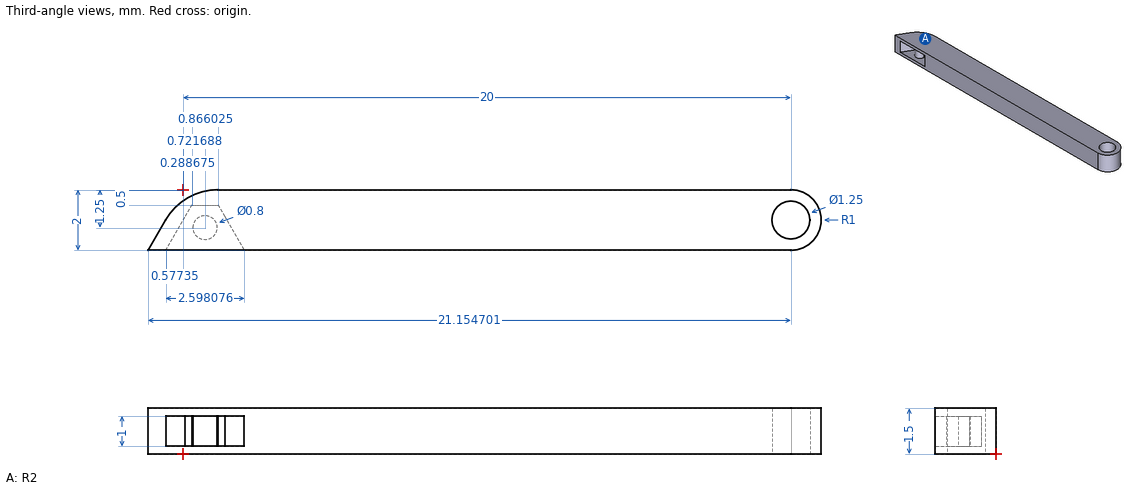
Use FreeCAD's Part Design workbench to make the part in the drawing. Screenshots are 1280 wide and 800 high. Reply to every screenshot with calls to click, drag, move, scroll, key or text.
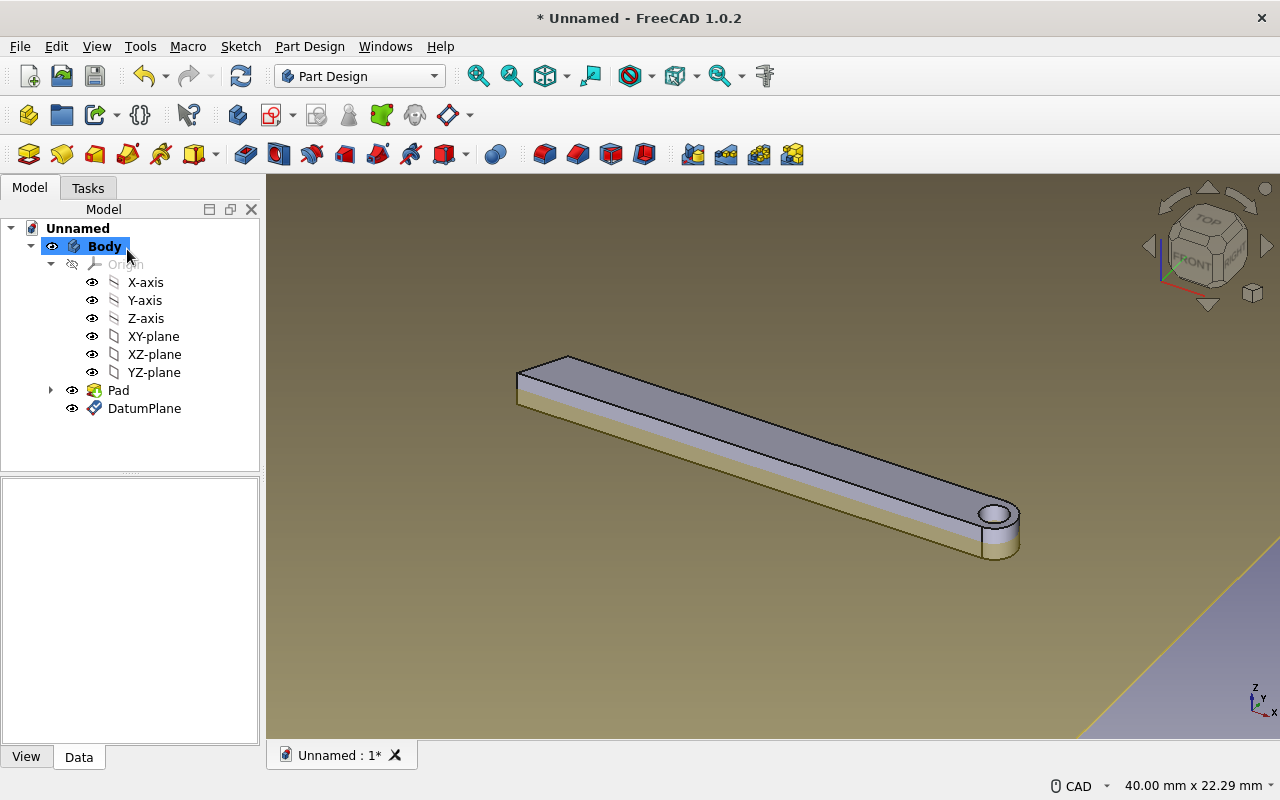
click(117, 408)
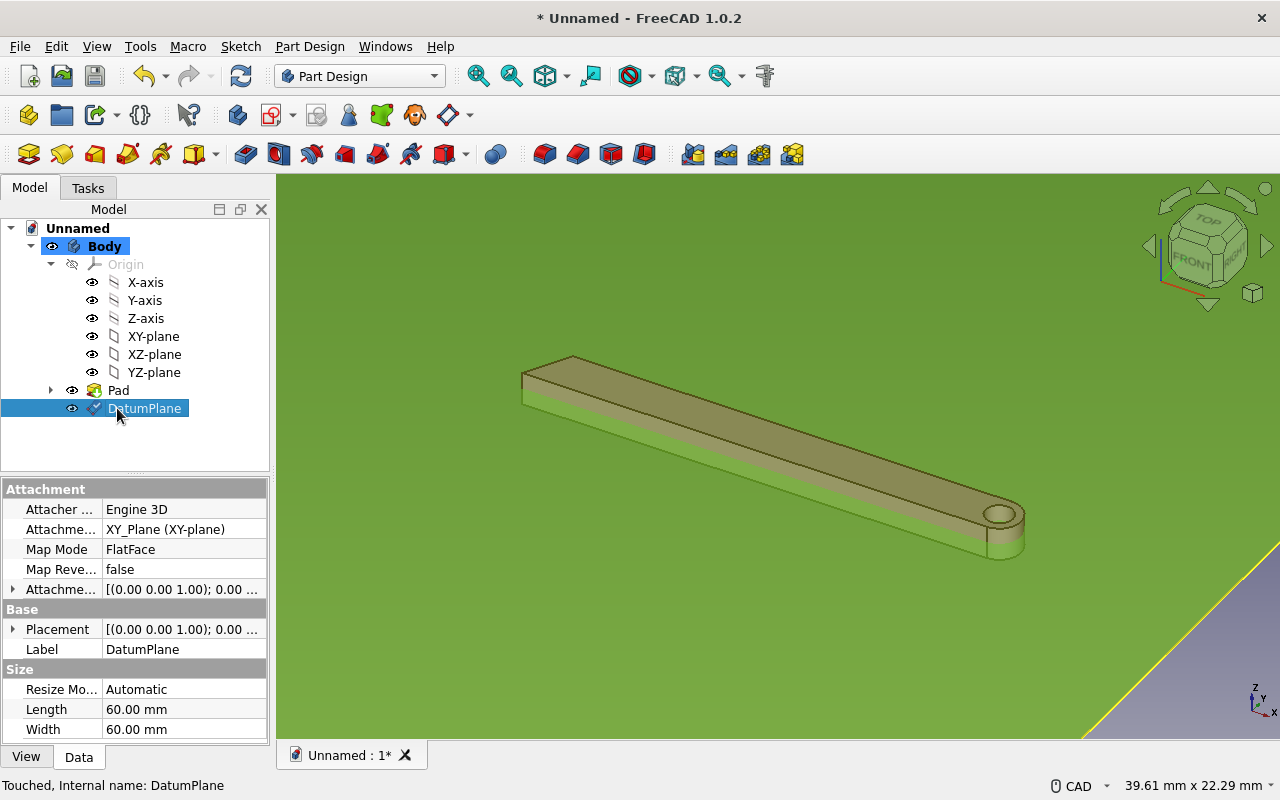
click(270, 116)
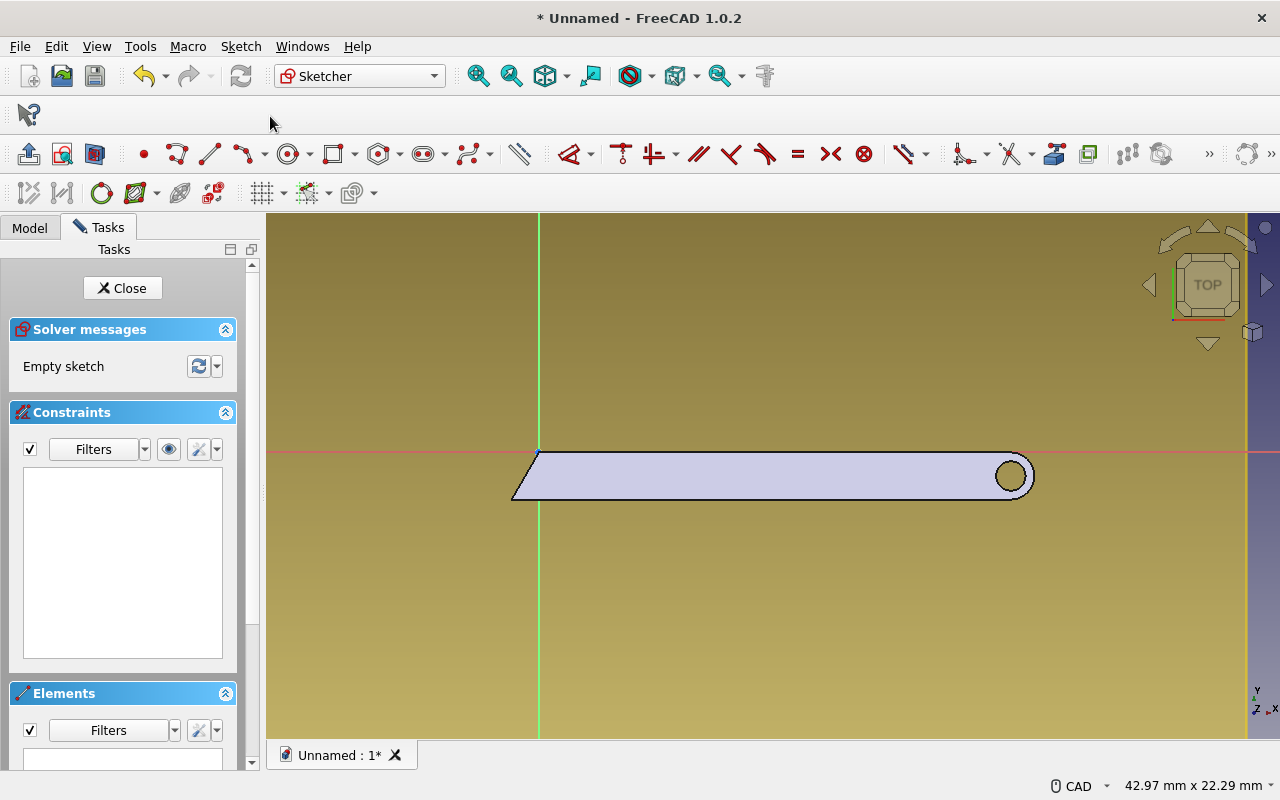
key(q)
key(s)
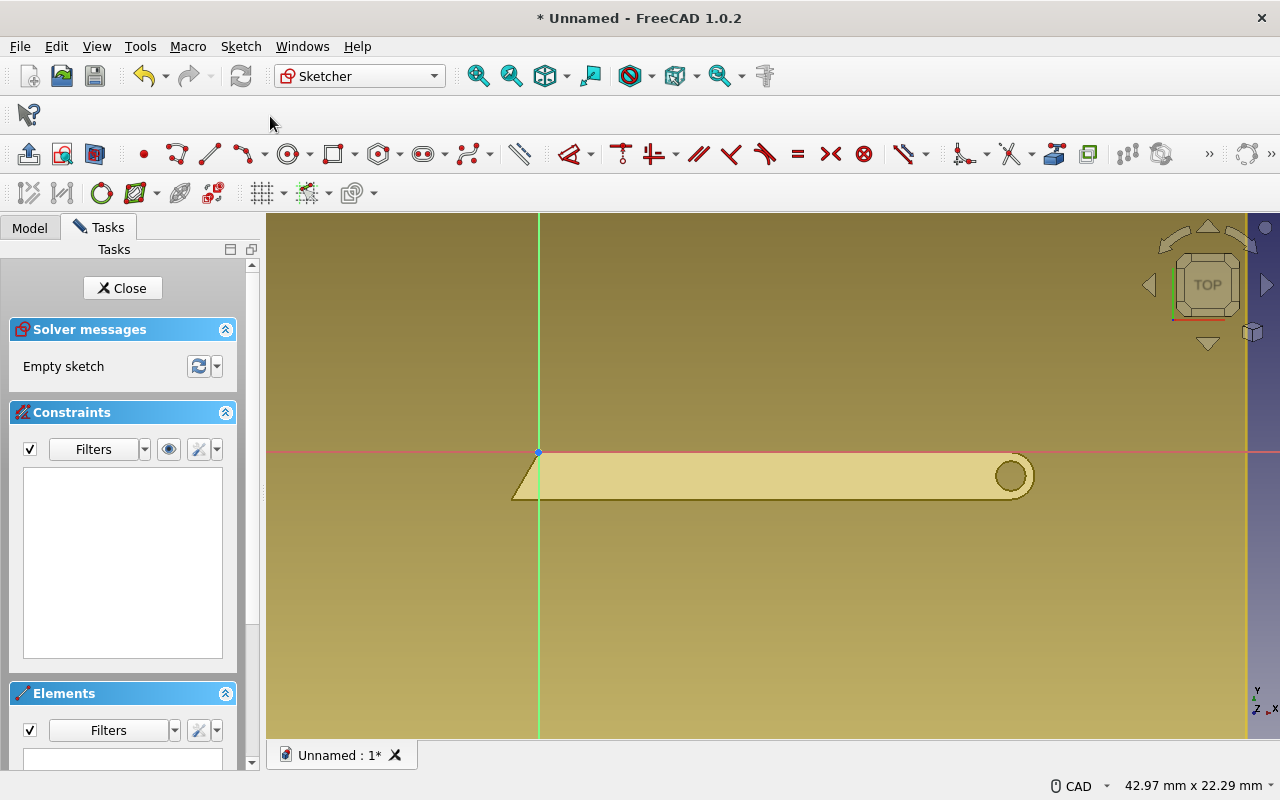
scroll(533, 476, up, 10)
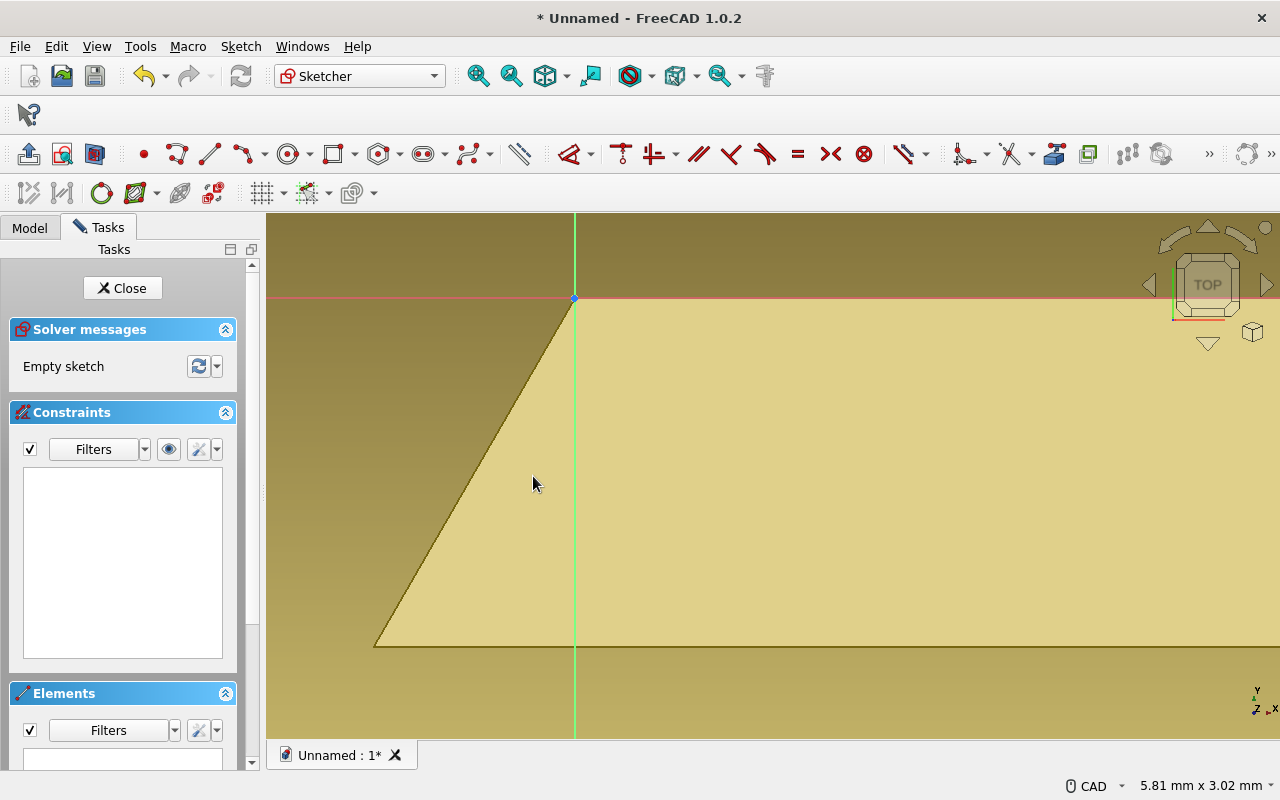
key(g)
key(m)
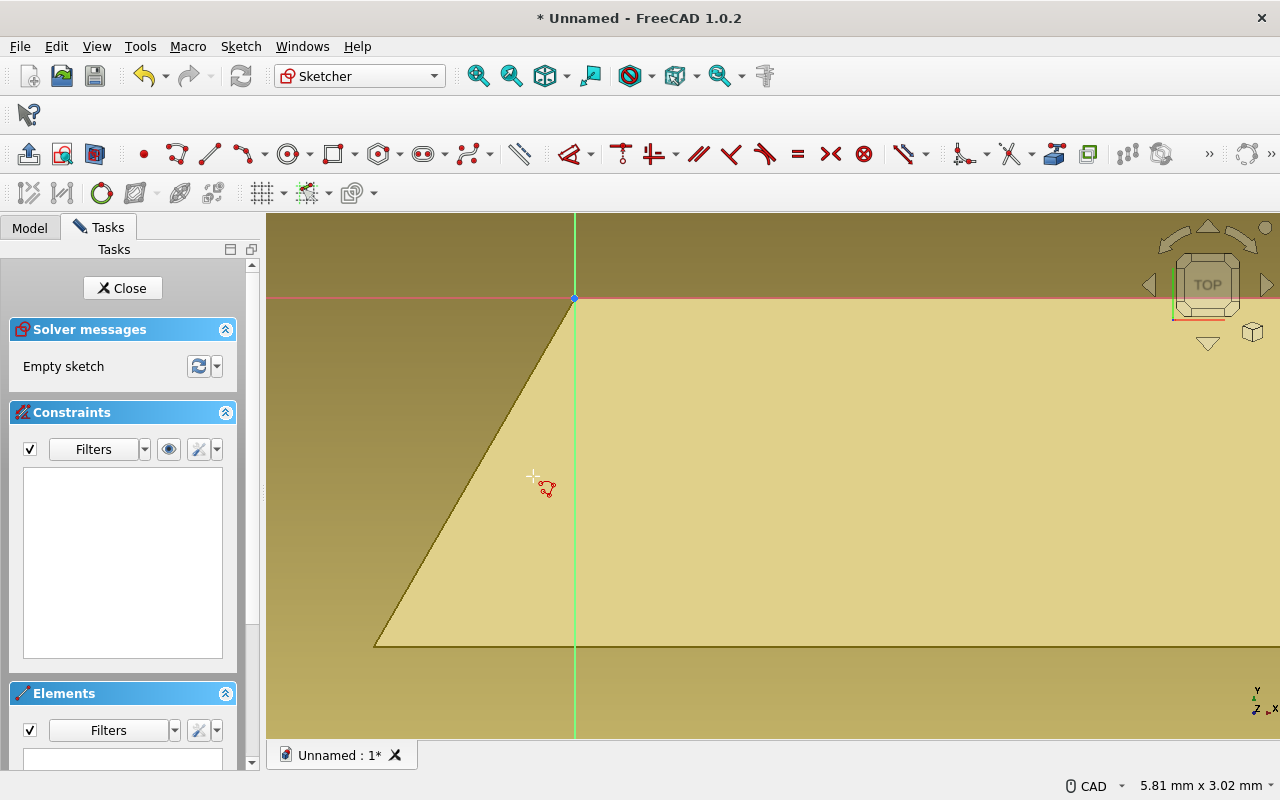
click(625, 386)
click(776, 386)
click(927, 647)
click(474, 647)
click(625, 387)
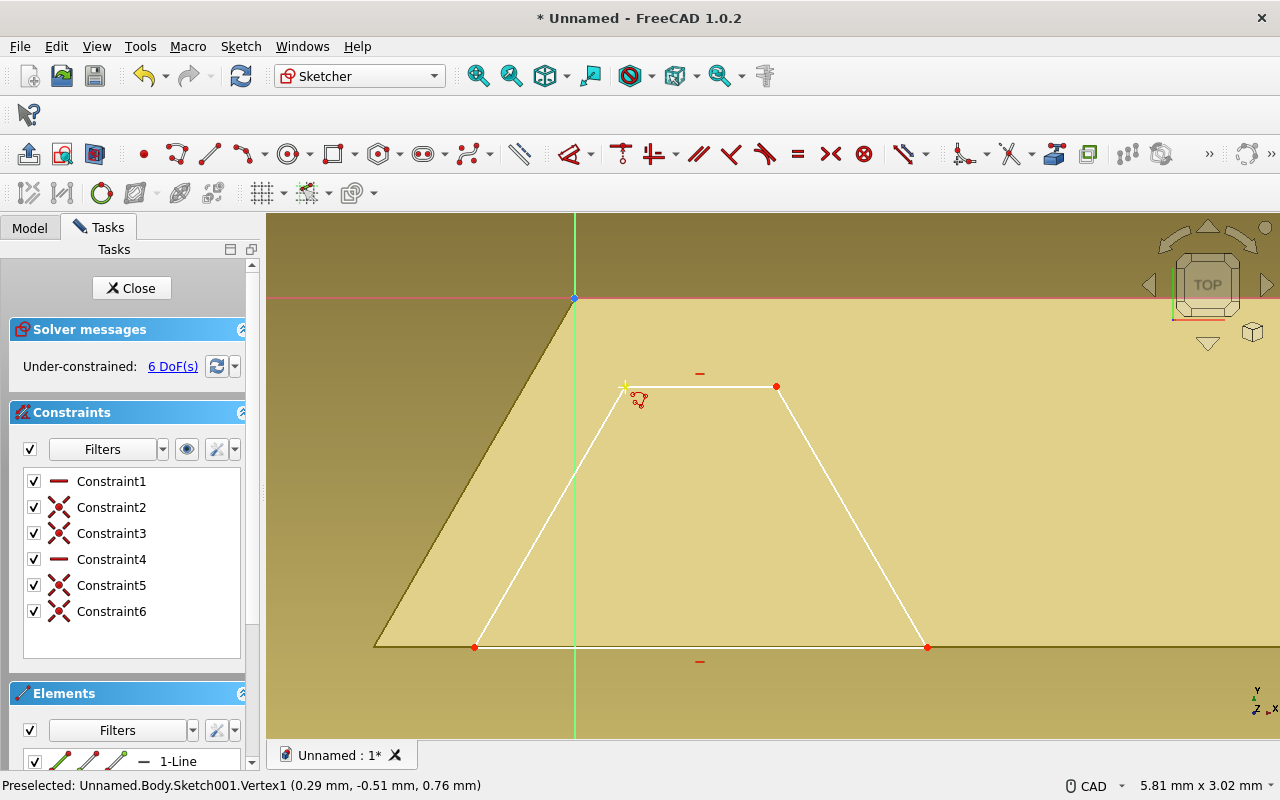
click(288, 154)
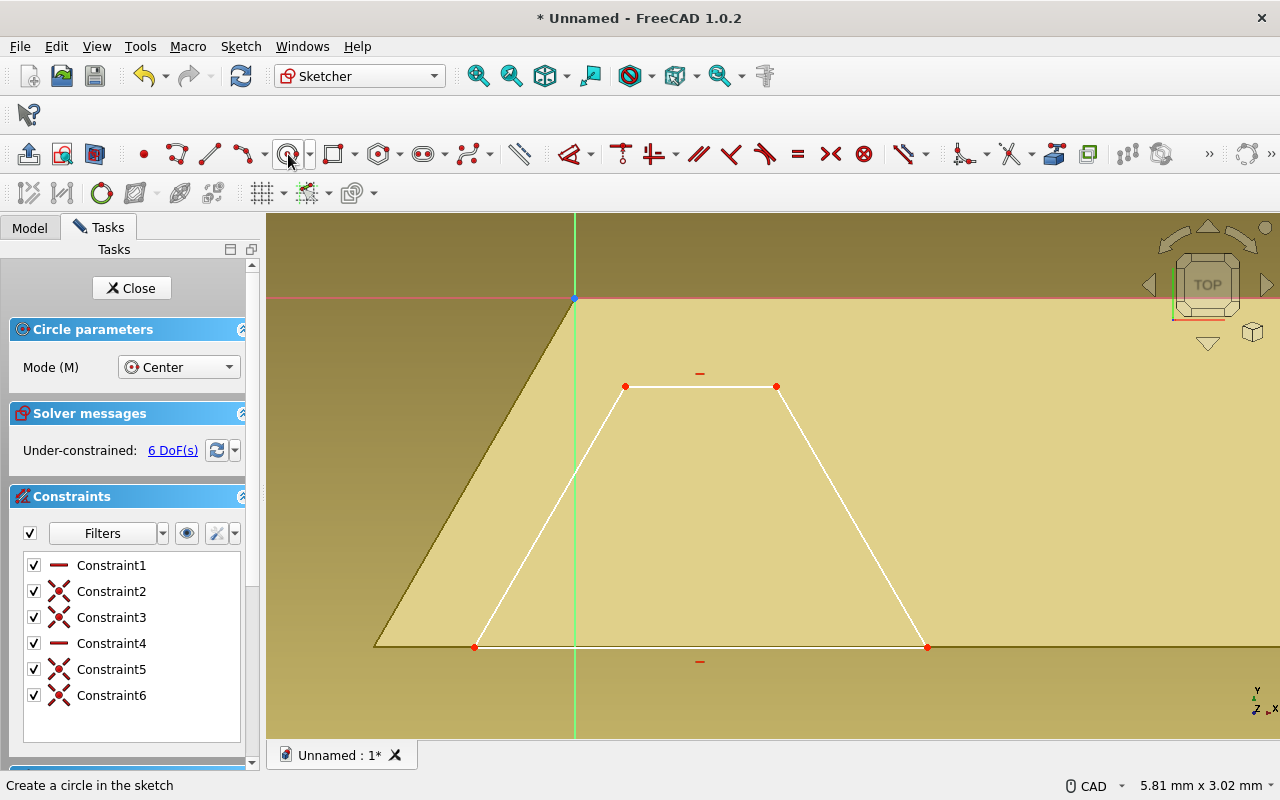
click(701, 516)
move(750, 467)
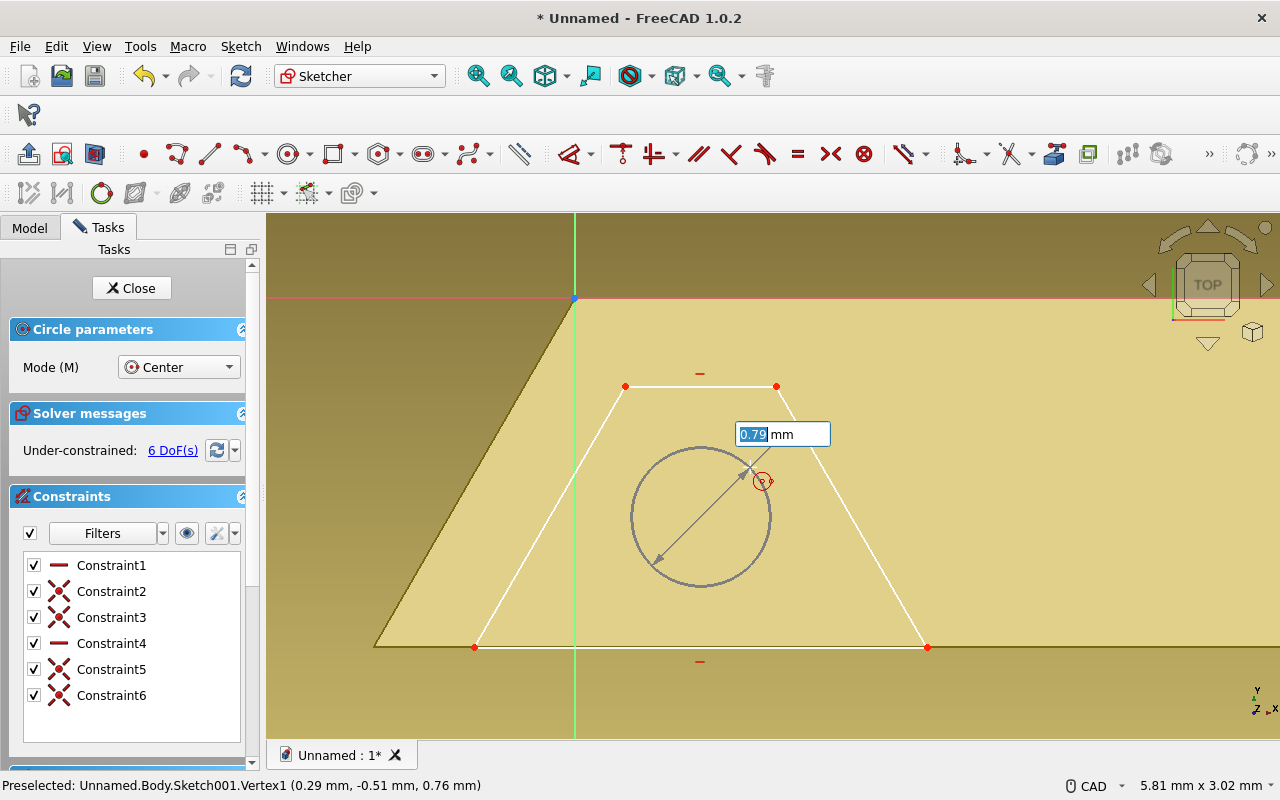
text(0.8)
key(Return)
key(Escape)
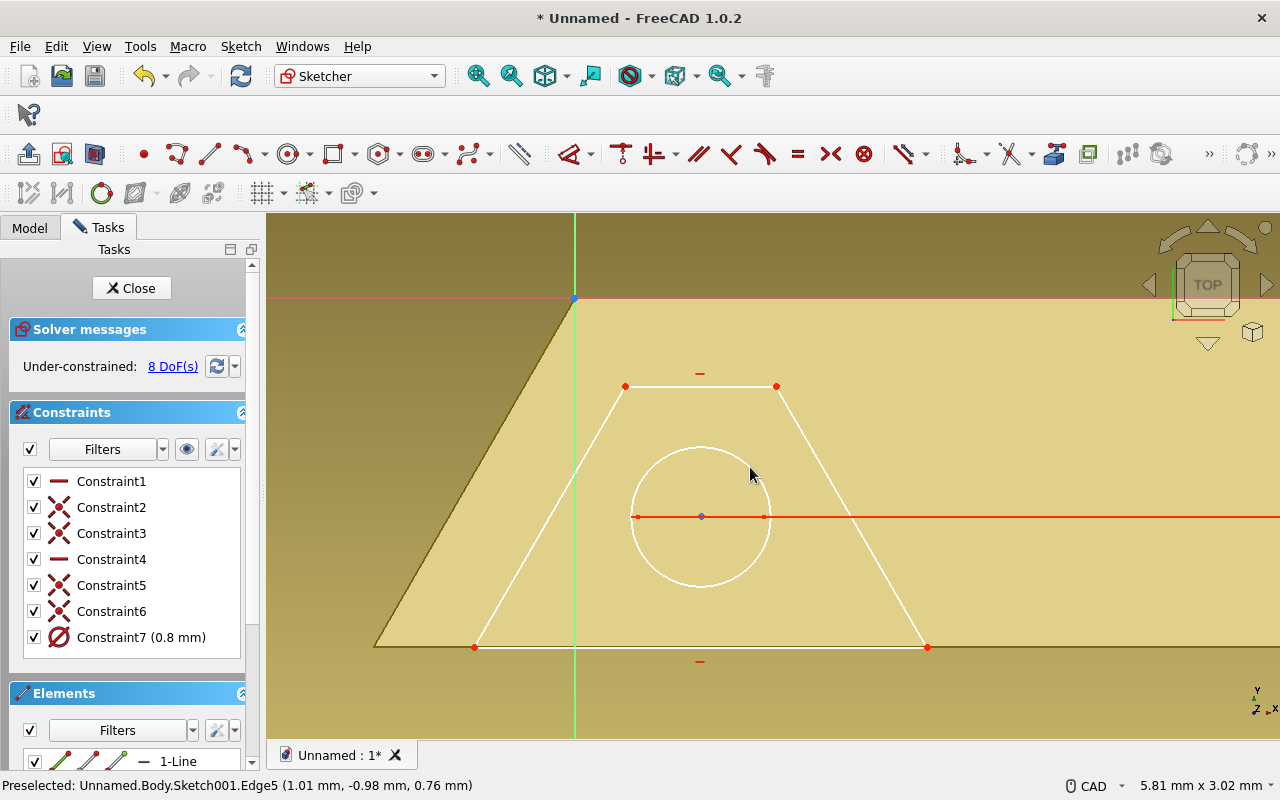
click(568, 154)